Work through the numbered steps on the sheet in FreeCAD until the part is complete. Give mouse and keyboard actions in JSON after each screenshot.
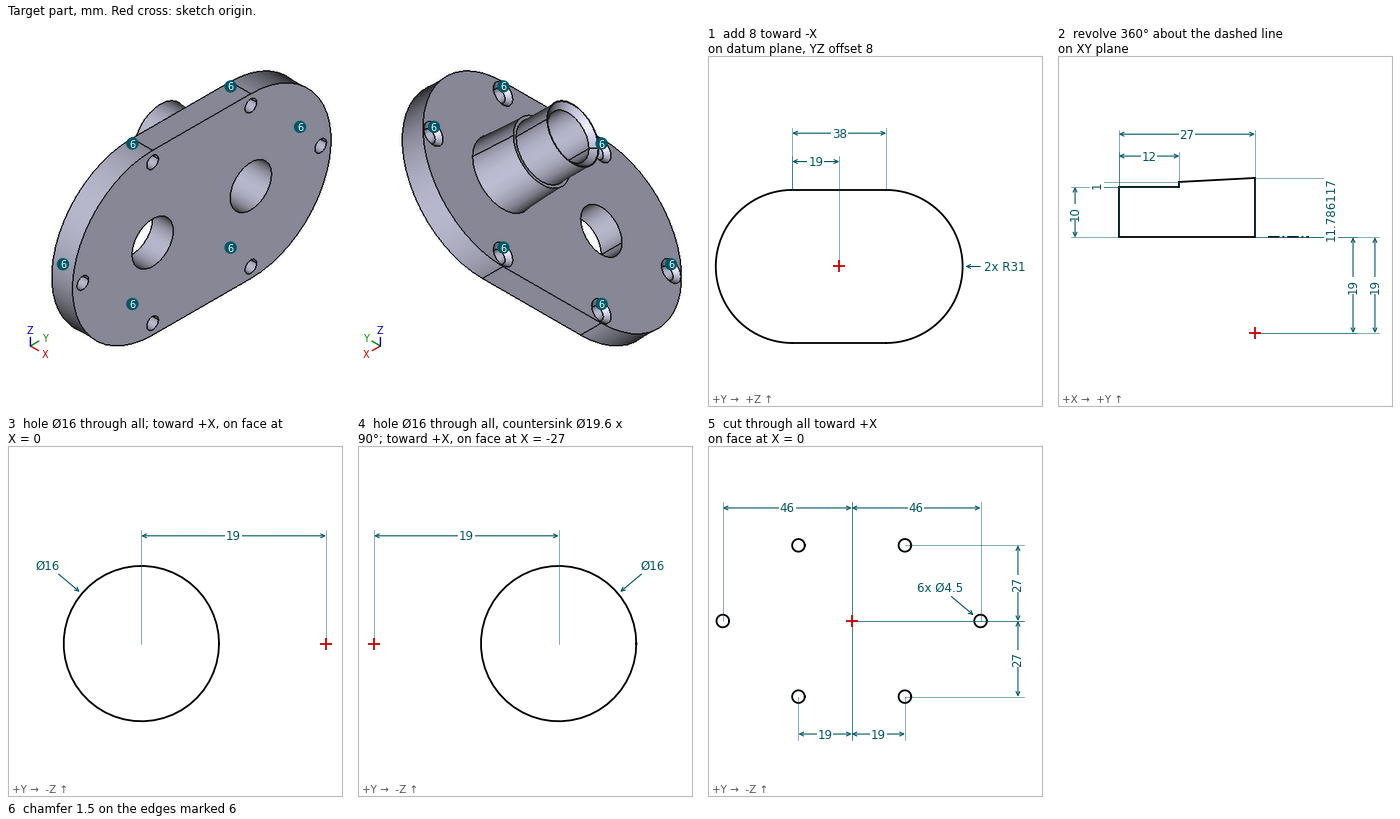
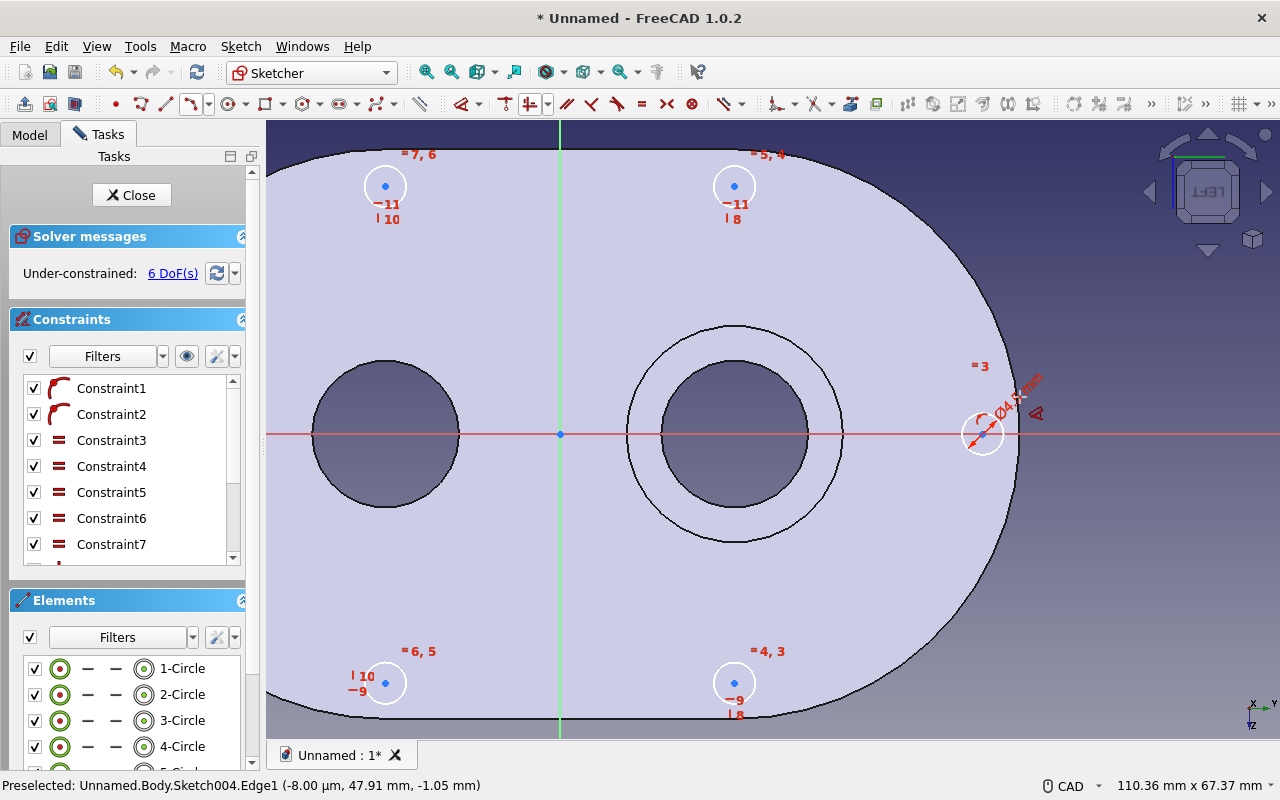
{"action": "left_click", "coordinate": [983, 434]}
{"action": "left_click", "coordinate": [772, 468]}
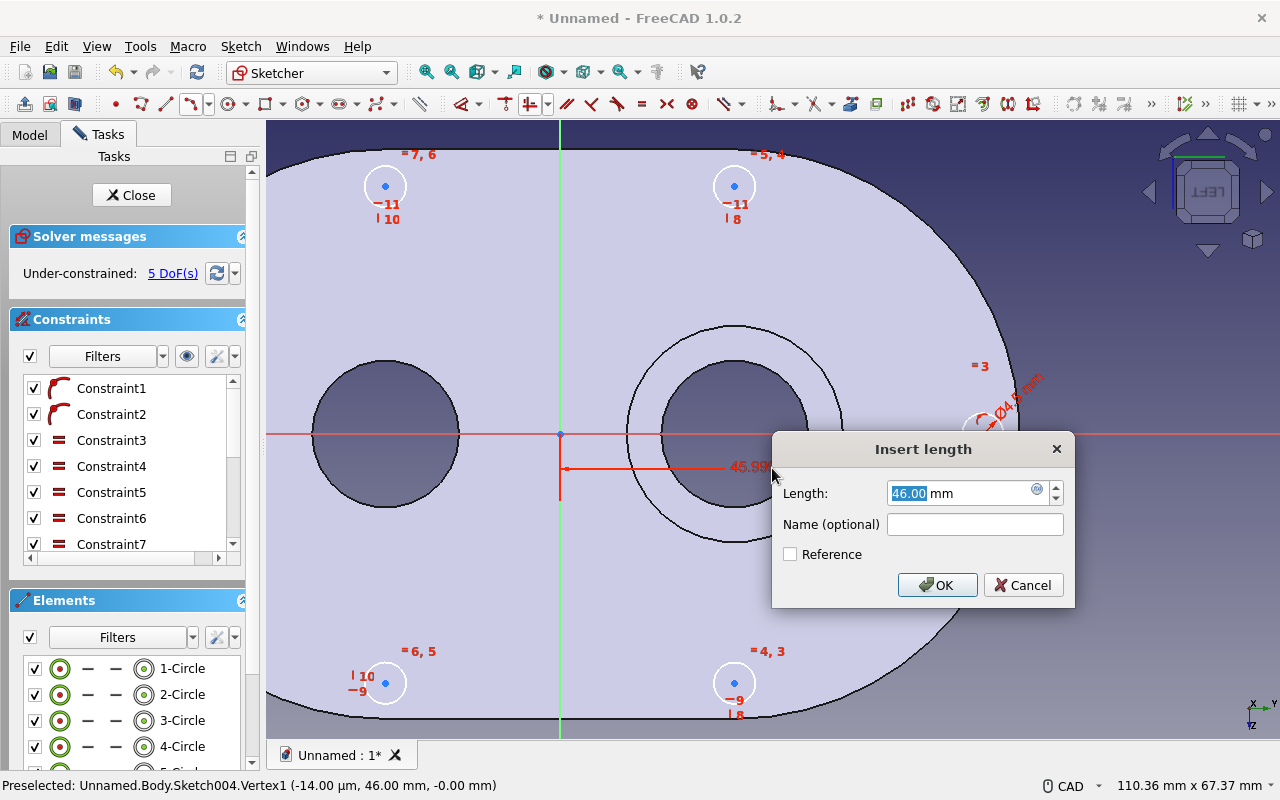
{"action": "type", "text": "46"}
{"action": "key", "text": "Return"}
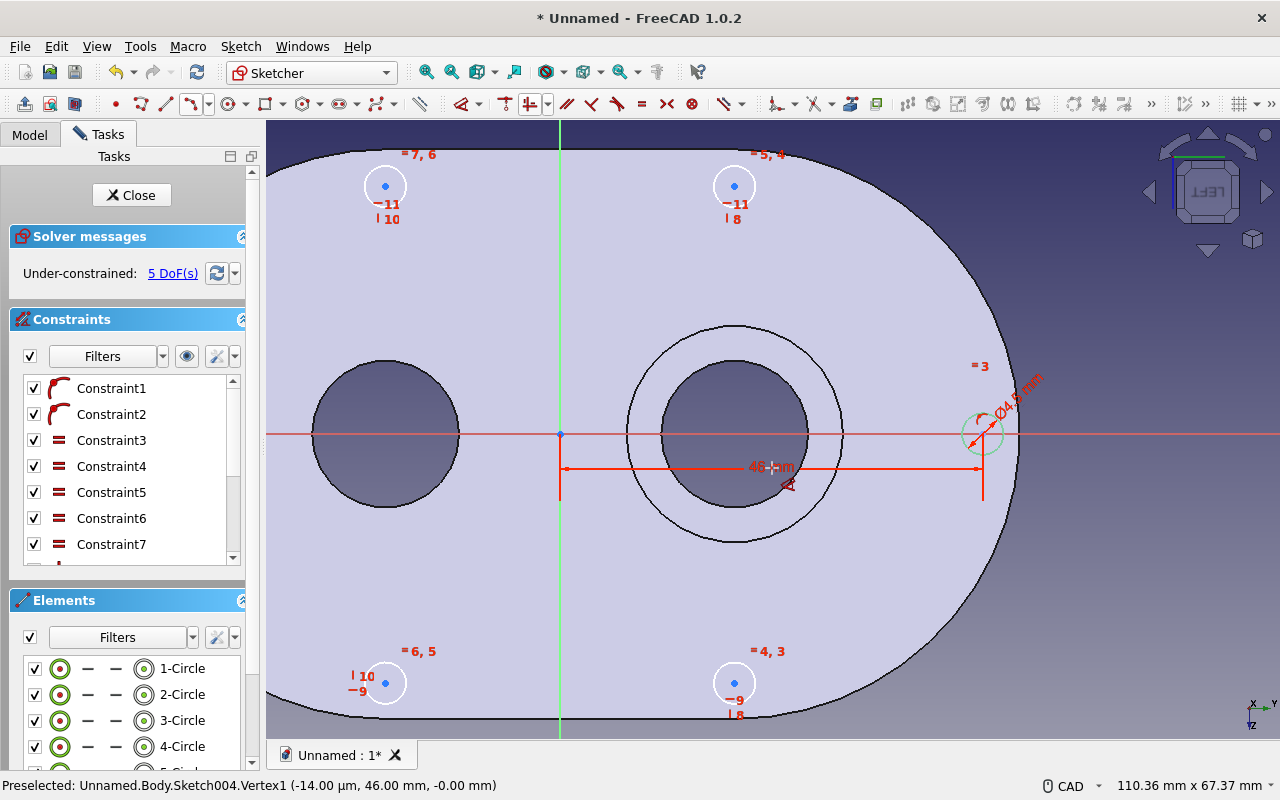
{"action": "left_click", "coordinate": [735, 683]}
{"action": "left_click", "coordinate": [647, 400]}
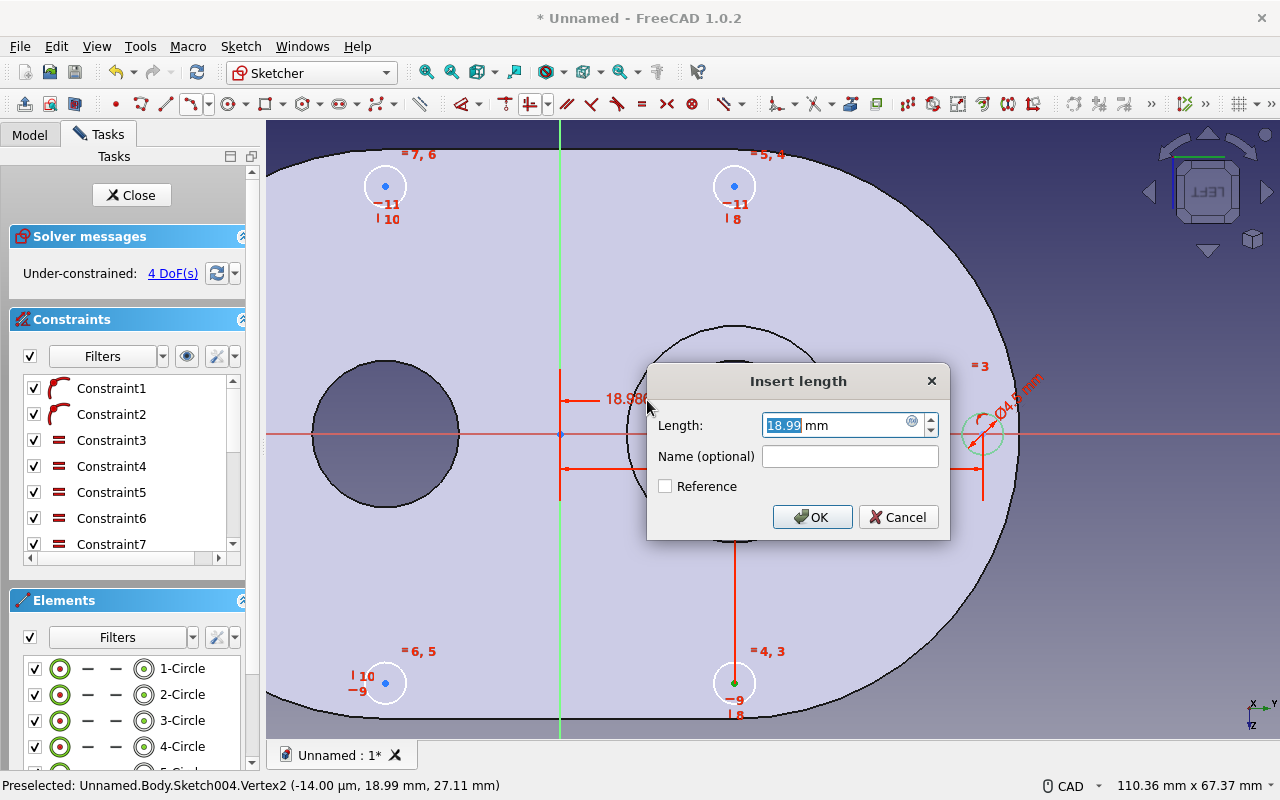
{"action": "type", "text": "19"}
{"action": "key", "text": "Return"}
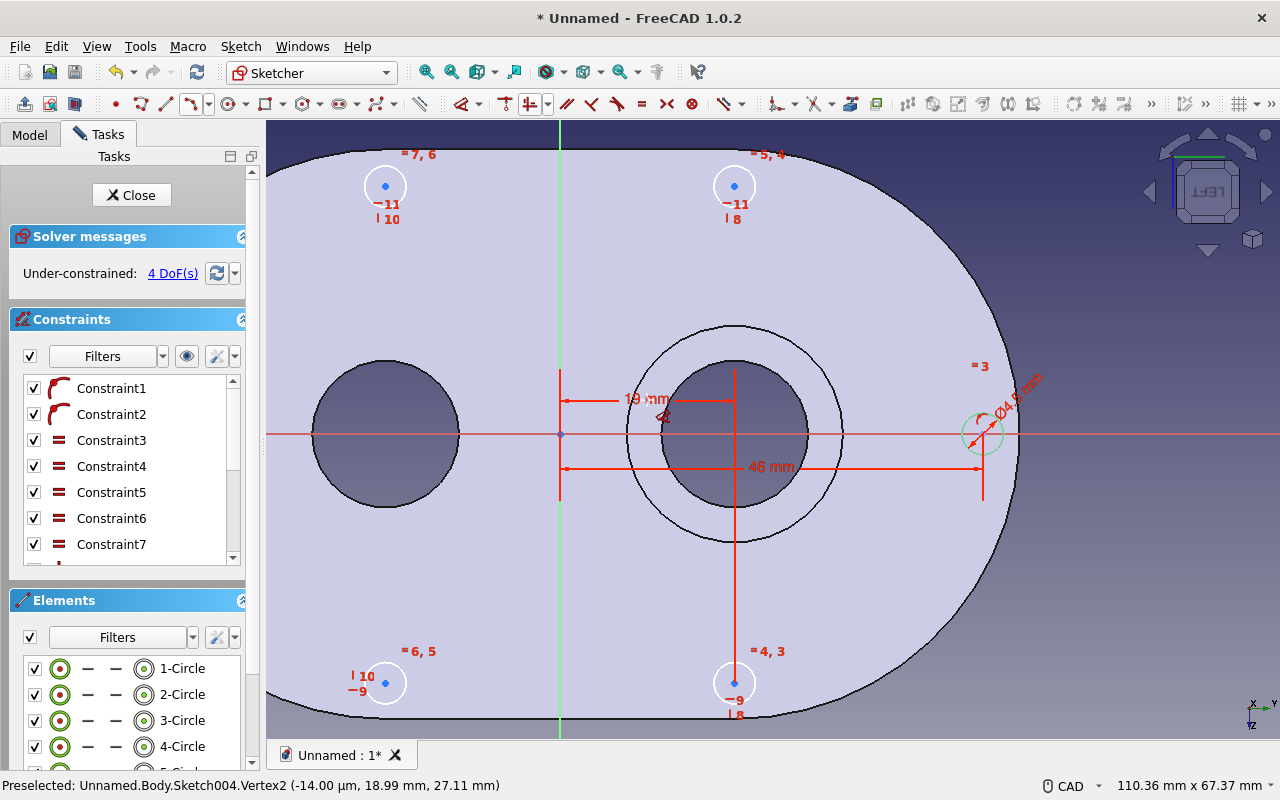
{"action": "left_click", "coordinate": [735, 683]}
{"action": "left_click", "coordinate": [769, 559]}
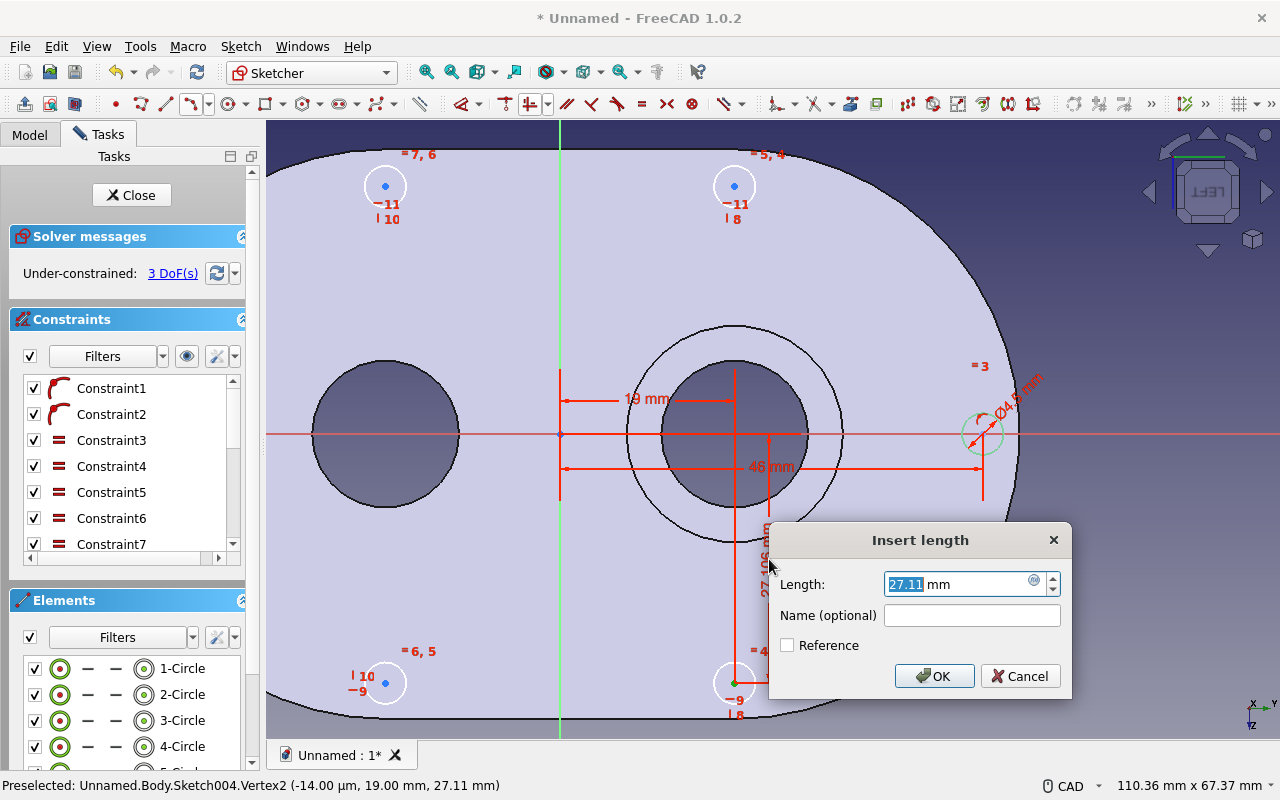
{"action": "type", "text": "27"}
{"action": "key", "text": "Return"}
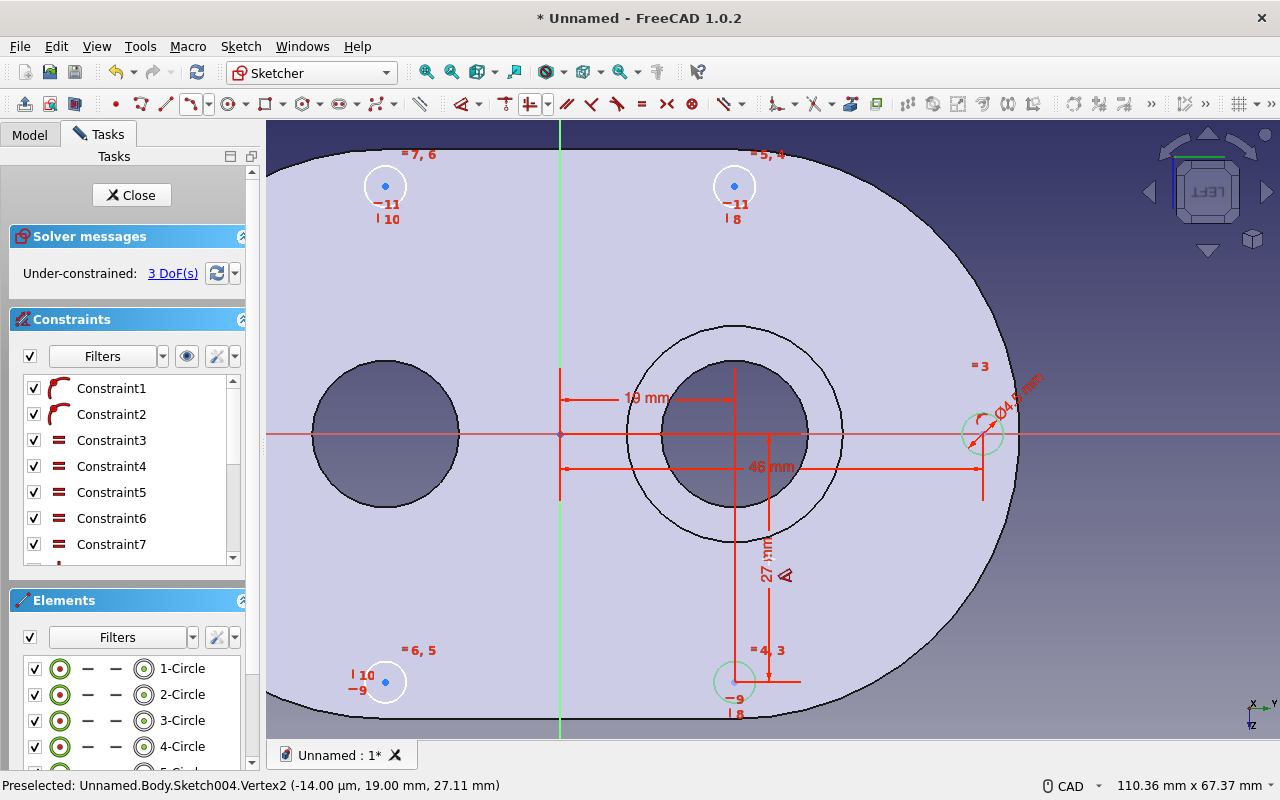
{"action": "left_click", "coordinate": [735, 187]}
{"action": "left_click", "coordinate": [769, 310]}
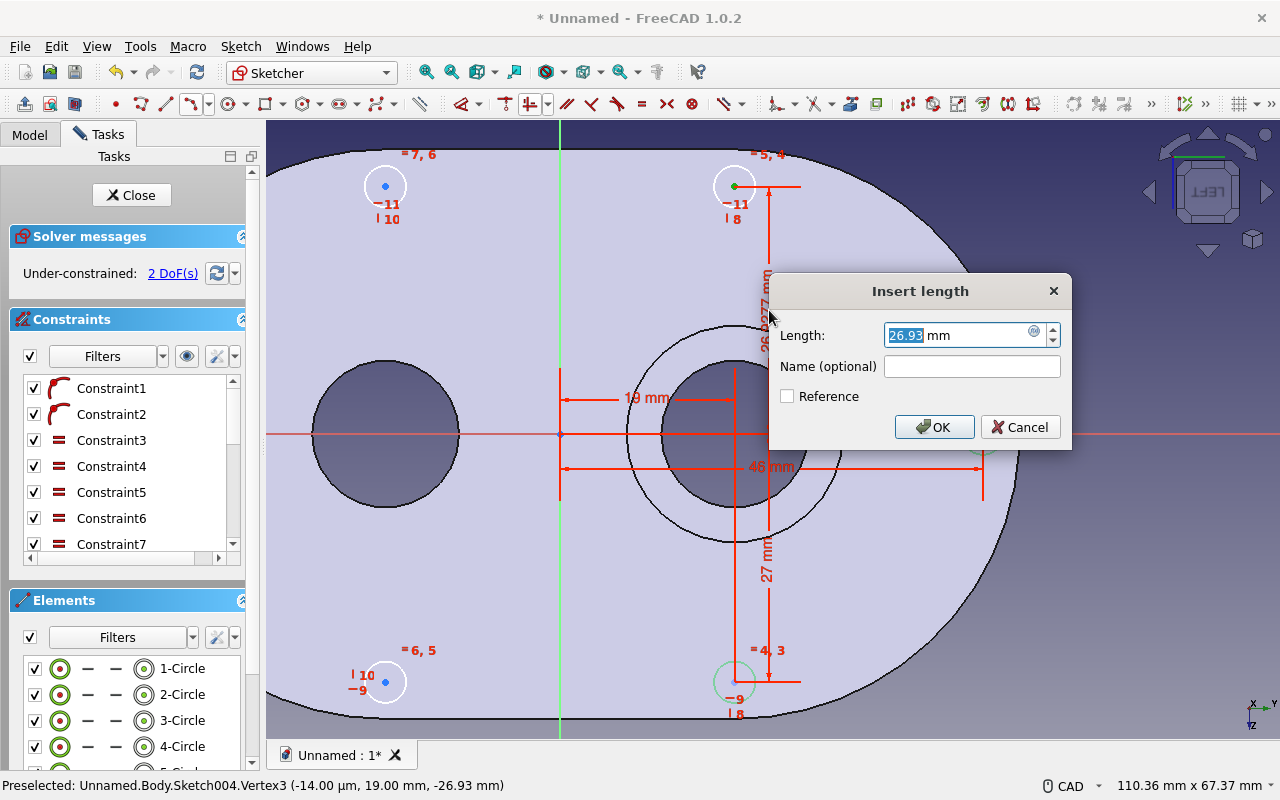
{"action": "type", "text": "27"}
{"action": "key", "text": "Return"}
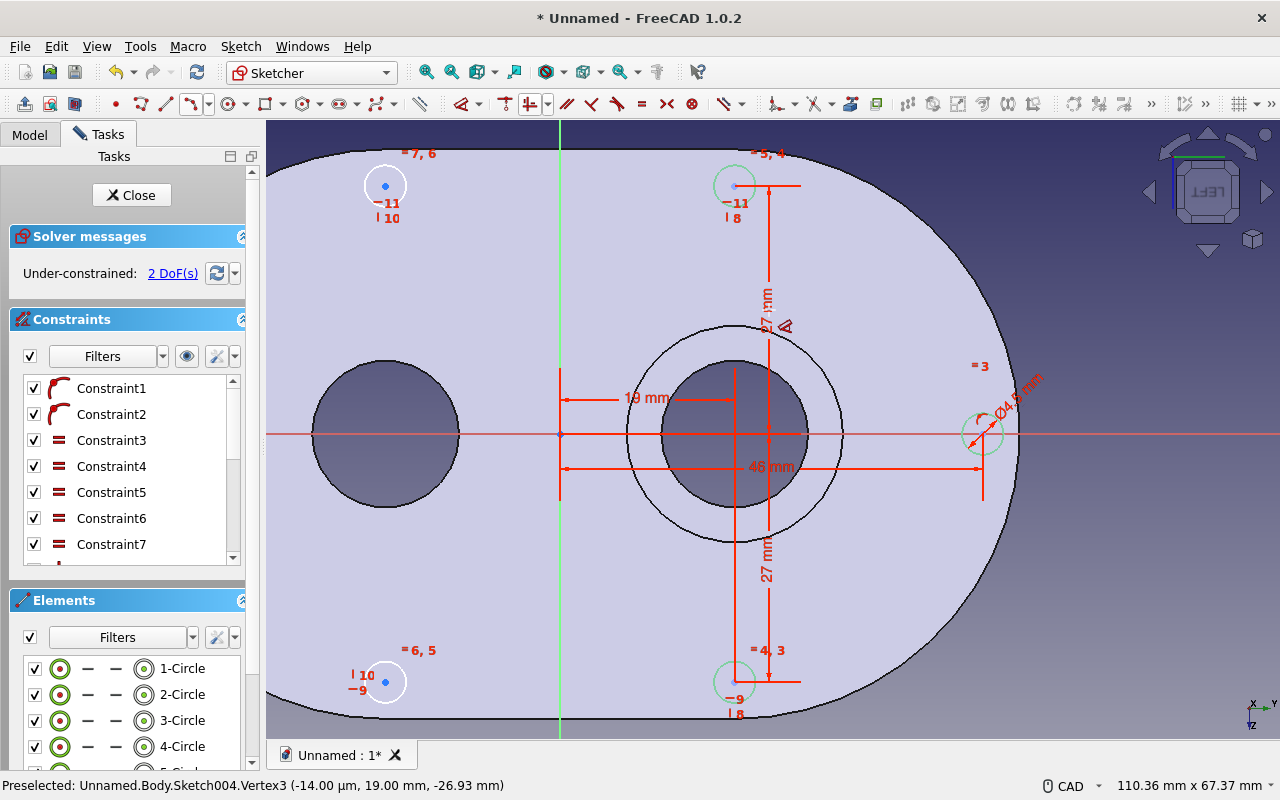
{"action": "left_click", "coordinate": [385, 682]}
{"action": "left_click", "coordinate": [473, 400]}